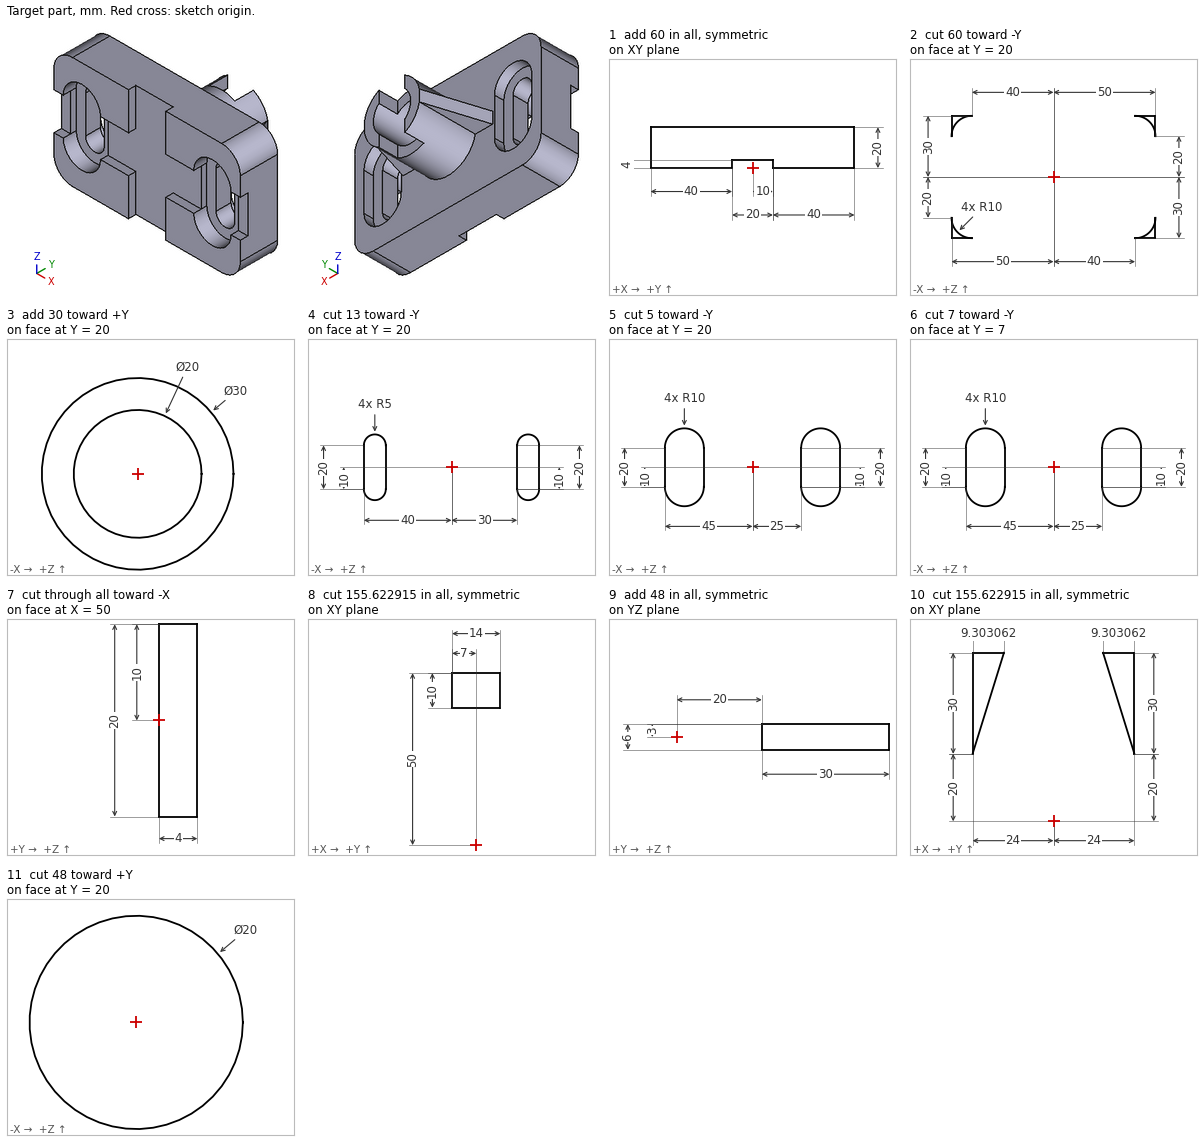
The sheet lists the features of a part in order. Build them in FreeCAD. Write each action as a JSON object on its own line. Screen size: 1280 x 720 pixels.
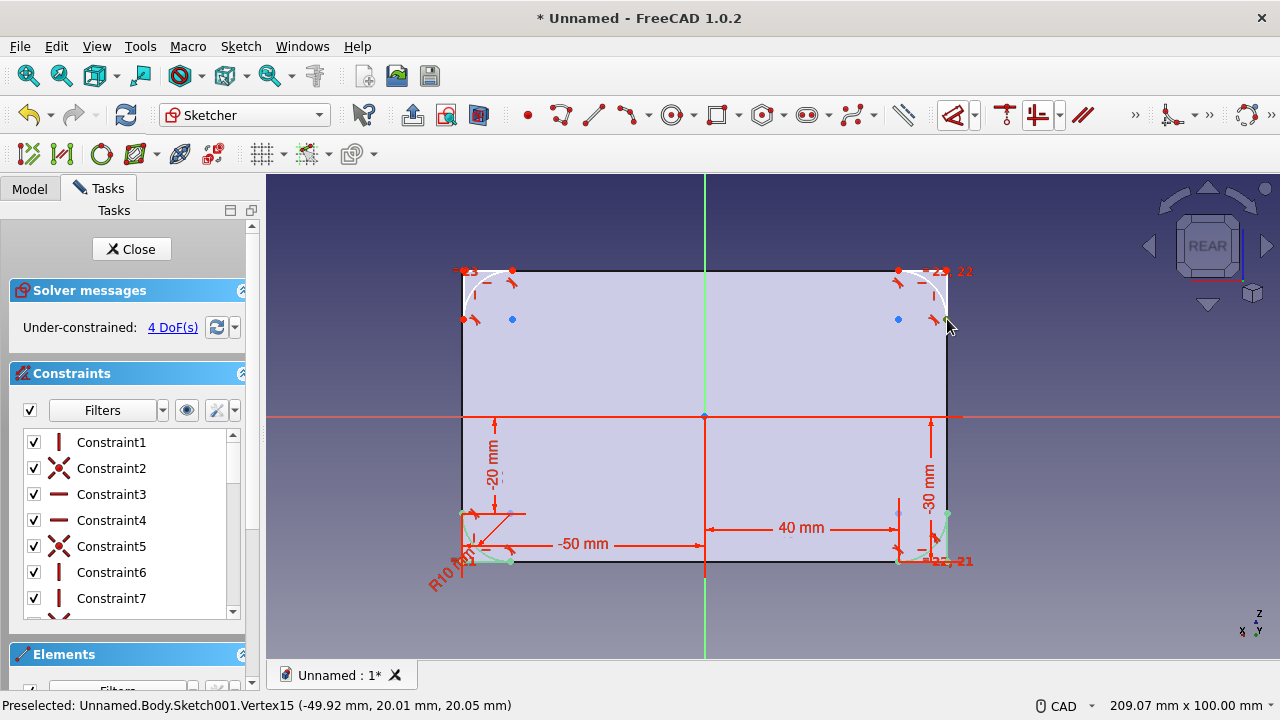
{"action": "key", "text": "l"}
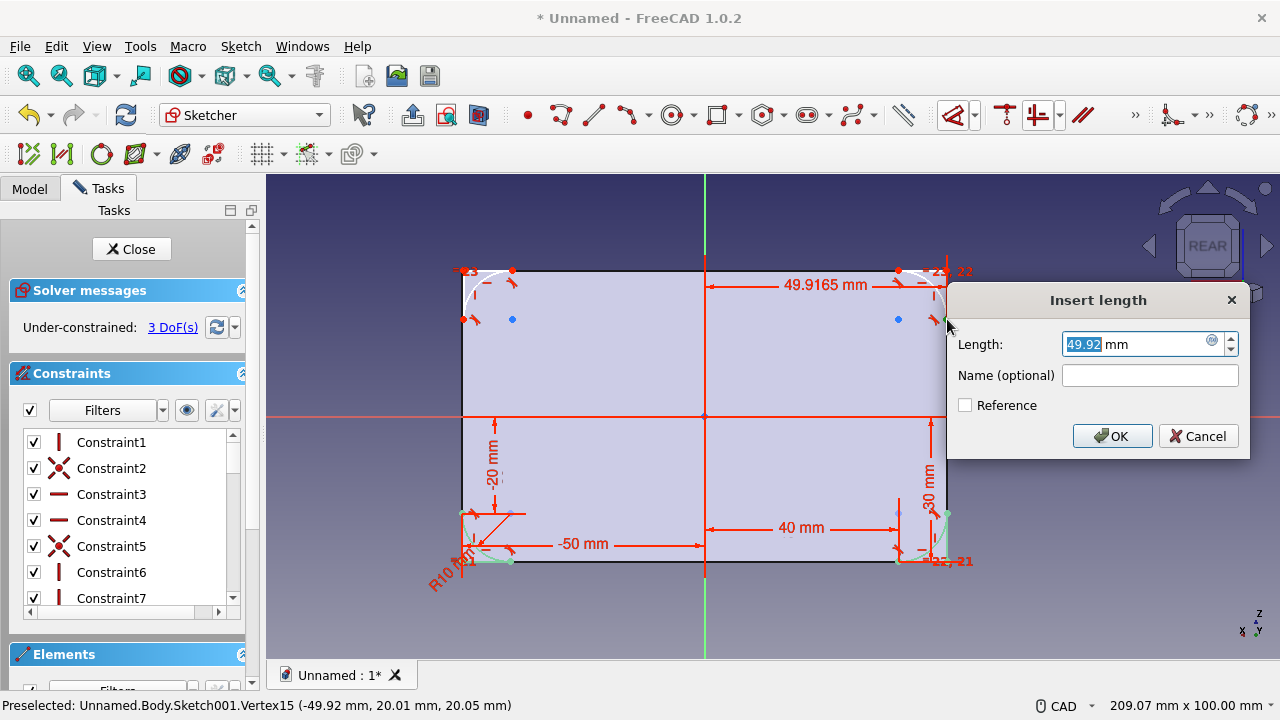
{"action": "type", "text": "50"}
{"action": "key", "text": "Return"}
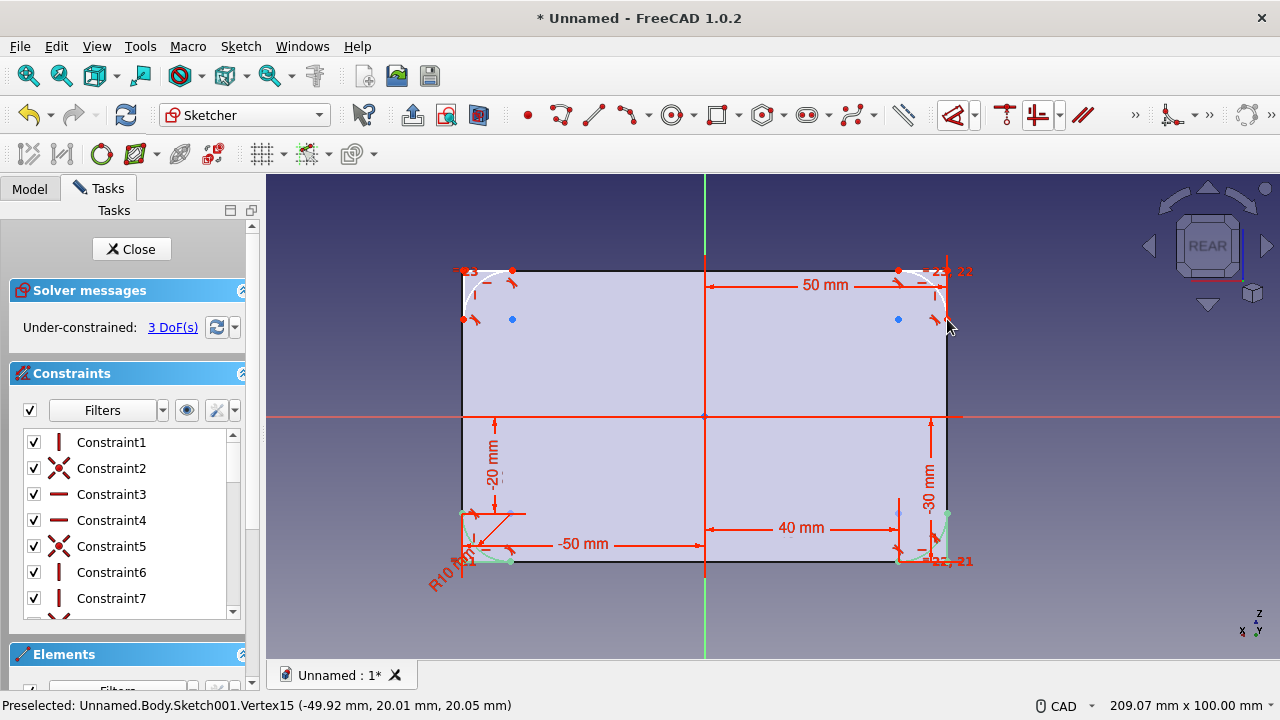
{"action": "left_click", "coordinate": [947, 319]}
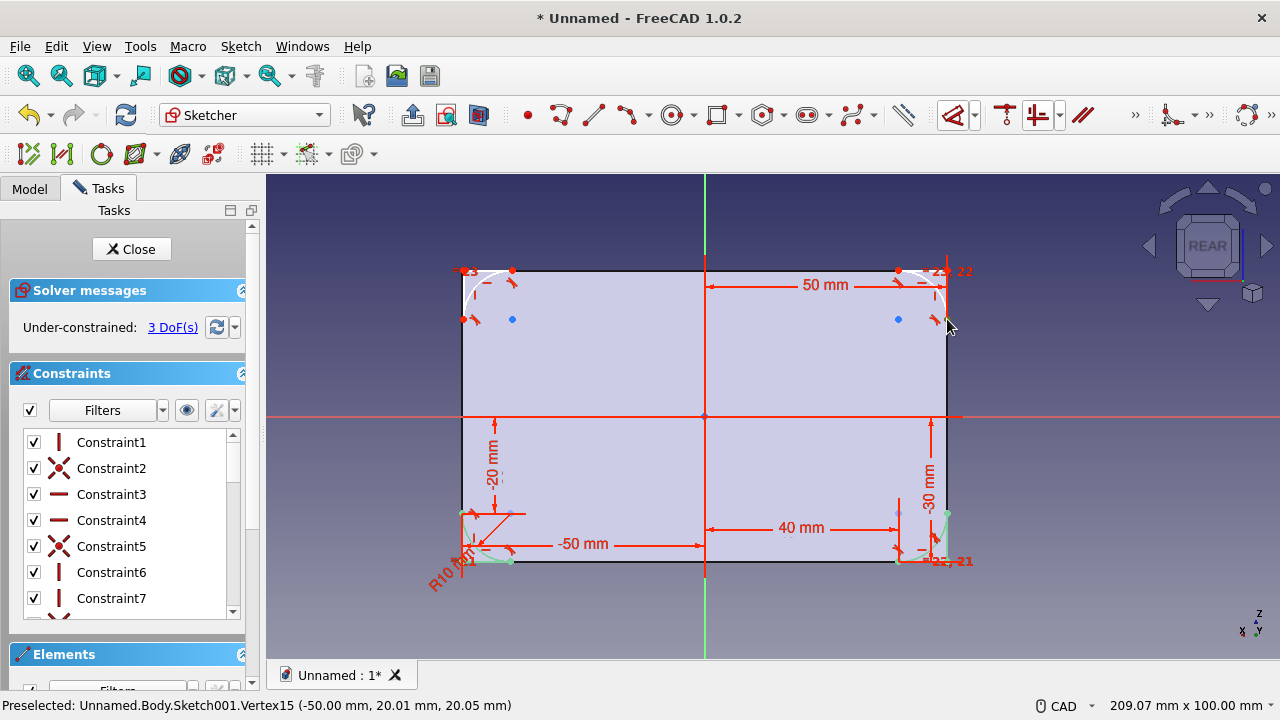
{"action": "key", "text": "i"}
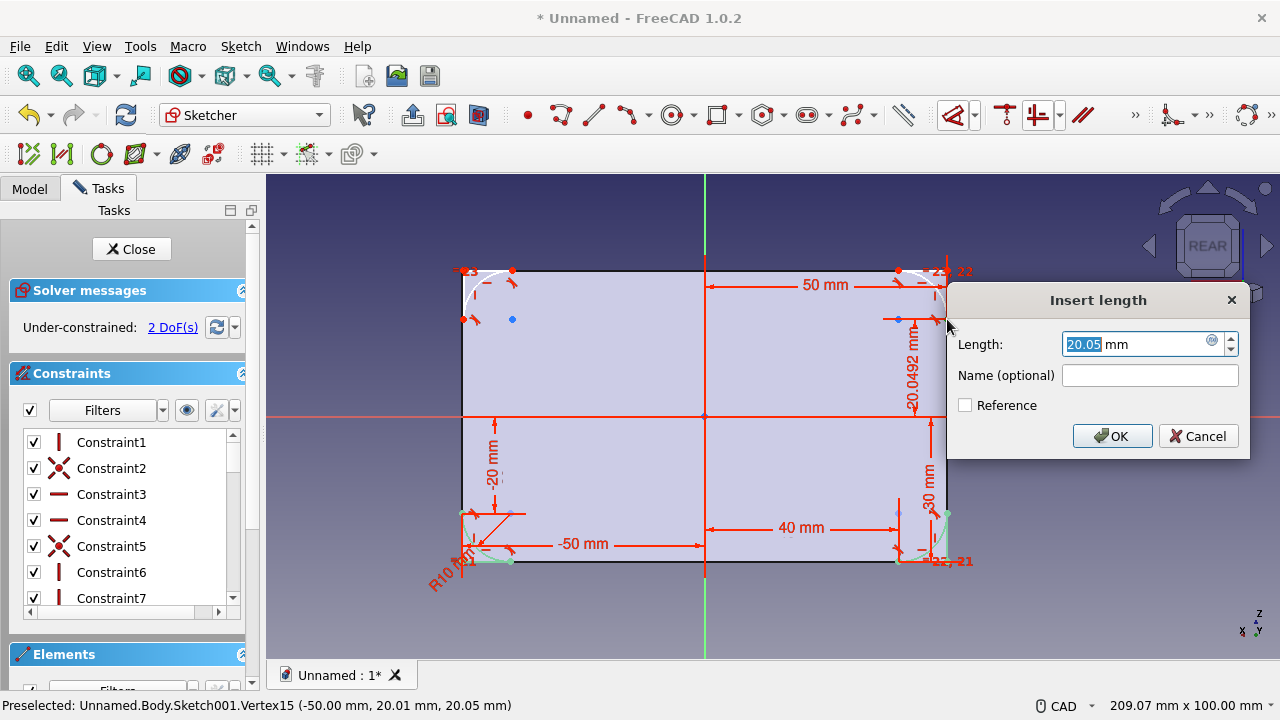
{"action": "type", "text": "20"}
{"action": "key", "text": "Return"}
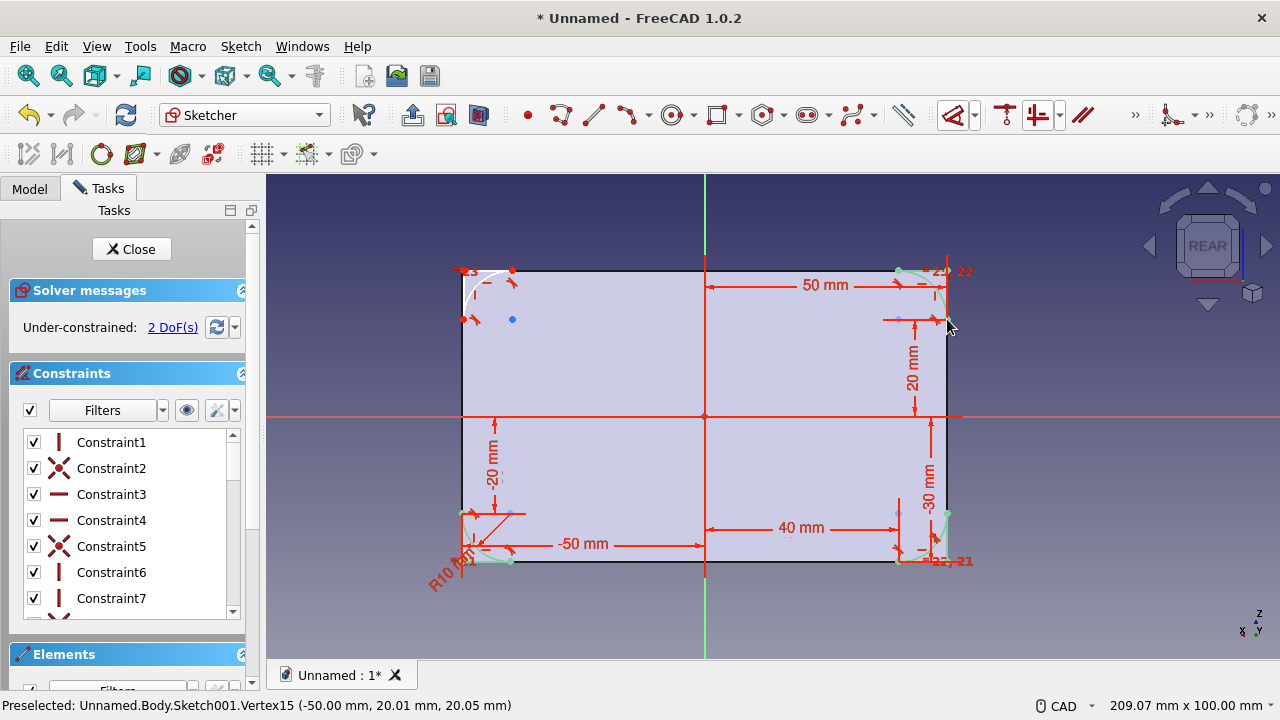
{"action": "left_click", "coordinate": [512, 271]}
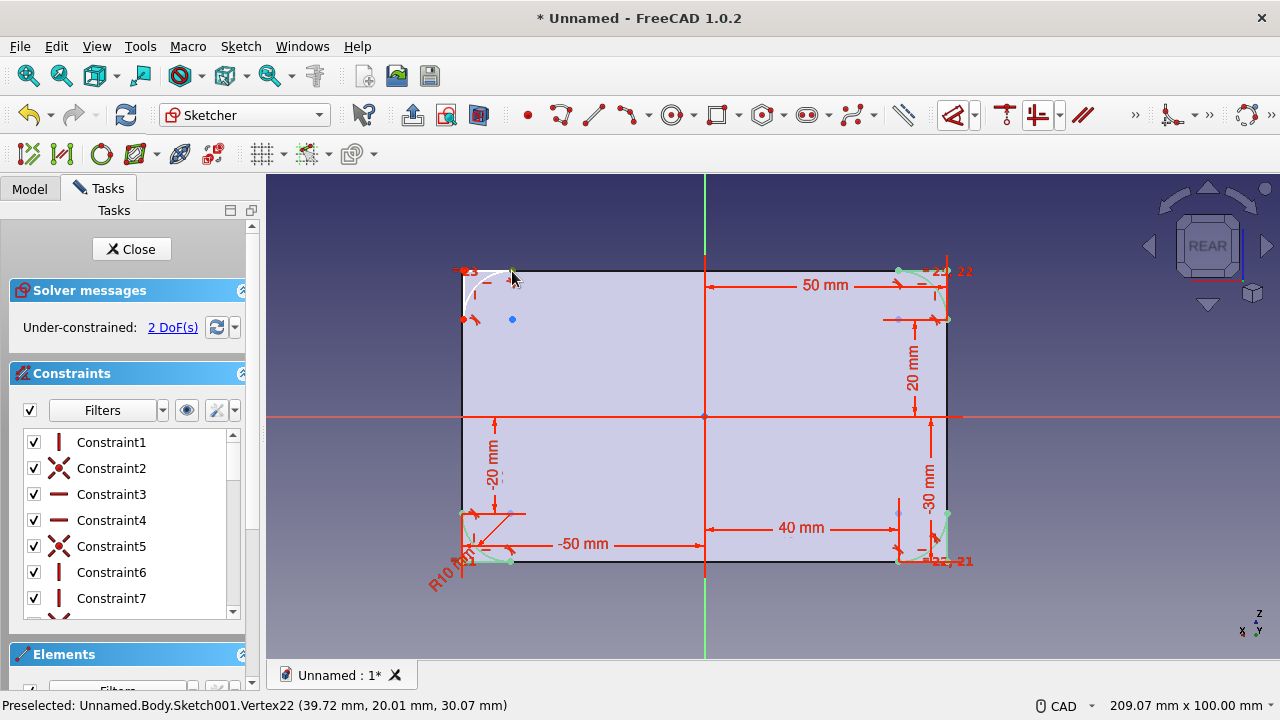
{"action": "left_click", "coordinate": [974, 116]}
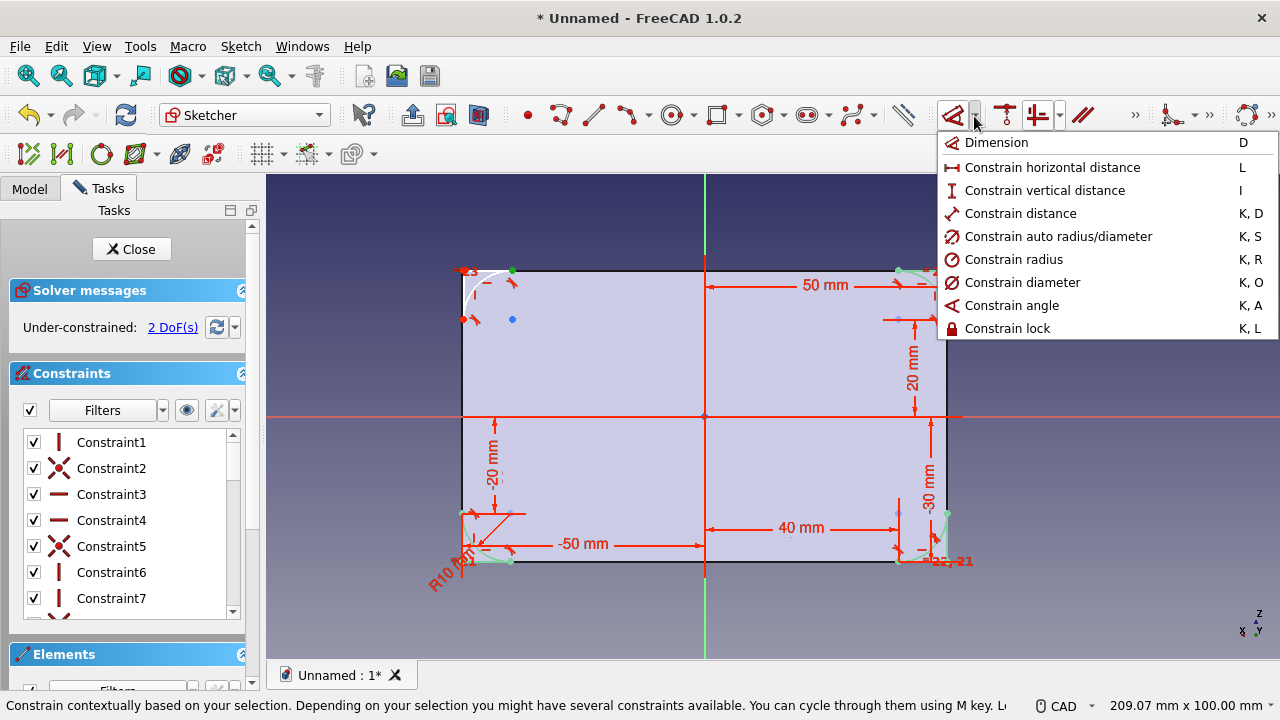
{"action": "left_click", "coordinate": [1108, 168]}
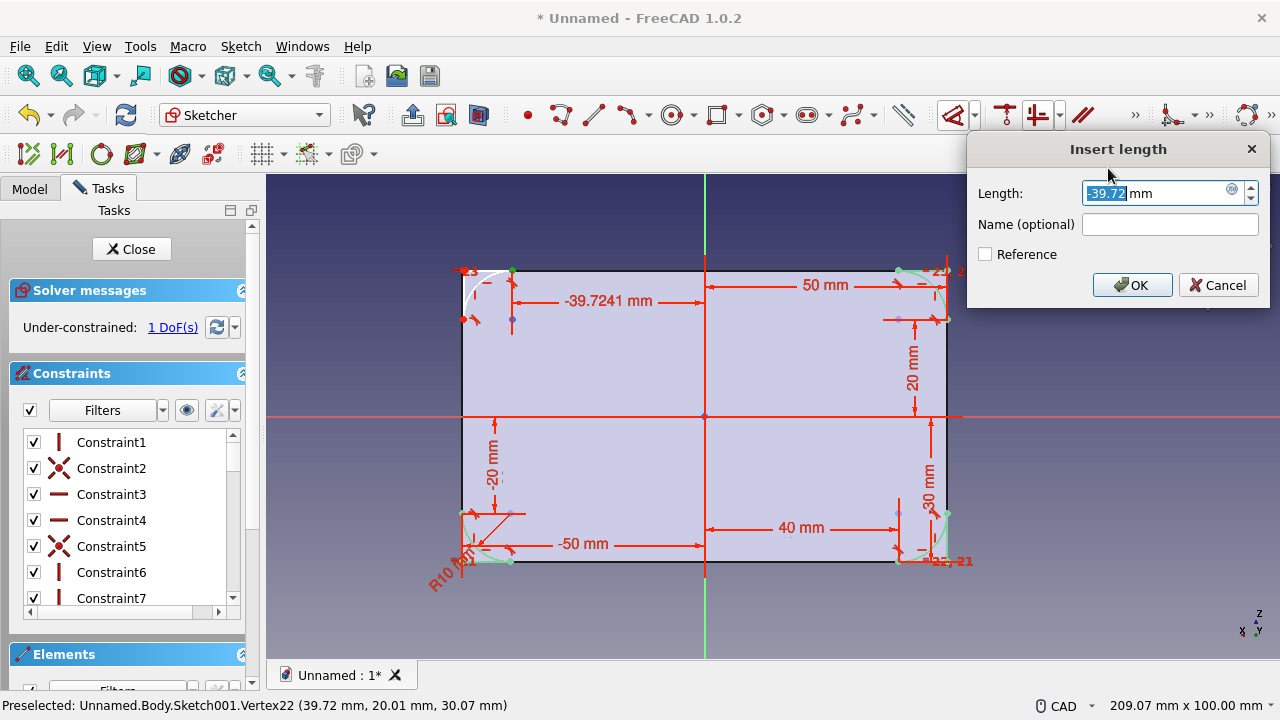
{"action": "type", "text": "-40"}
{"action": "key", "text": "Return"}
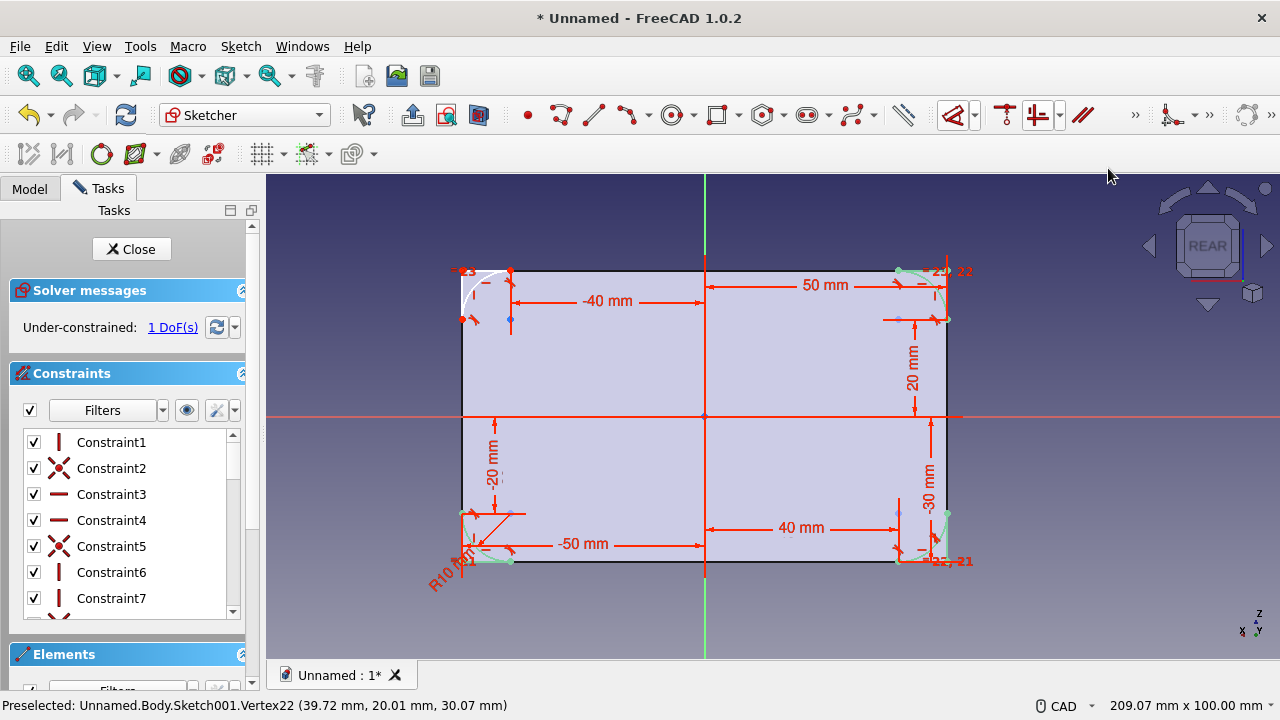
{"action": "left_click", "coordinate": [511, 271]}